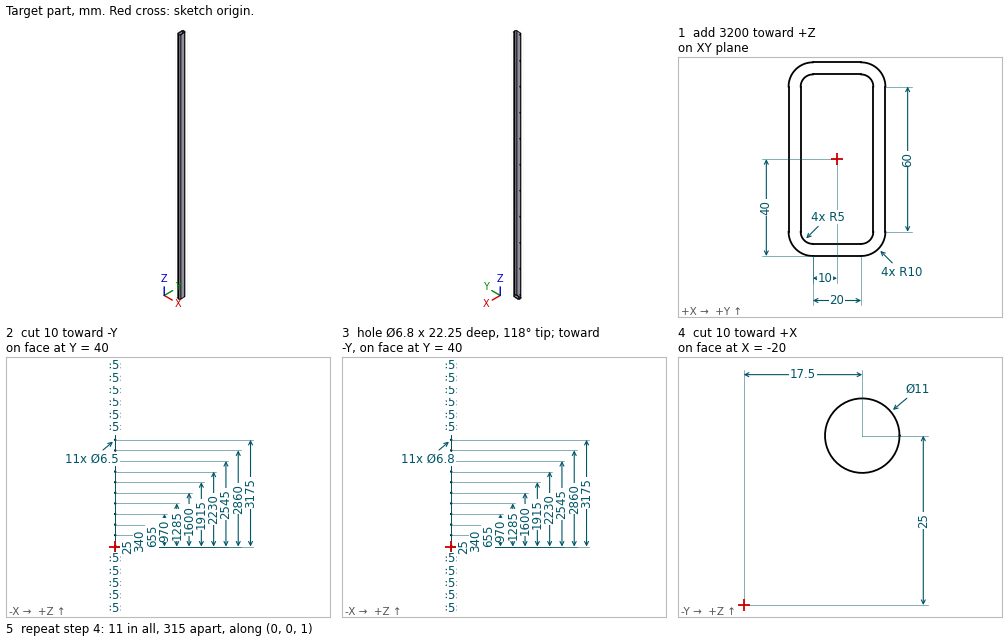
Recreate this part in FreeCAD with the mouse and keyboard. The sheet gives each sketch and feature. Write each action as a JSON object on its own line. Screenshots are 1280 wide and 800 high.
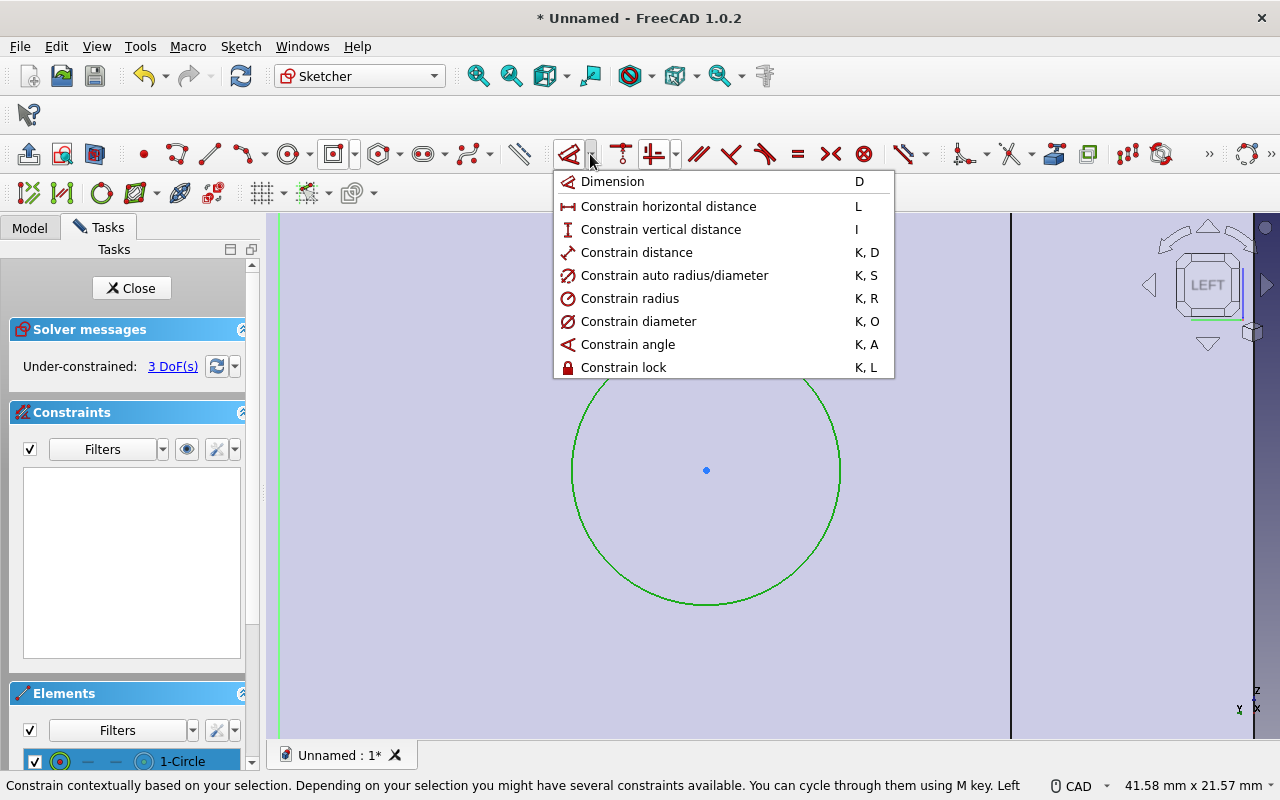
{"action": "left_click", "coordinate": [724, 322]}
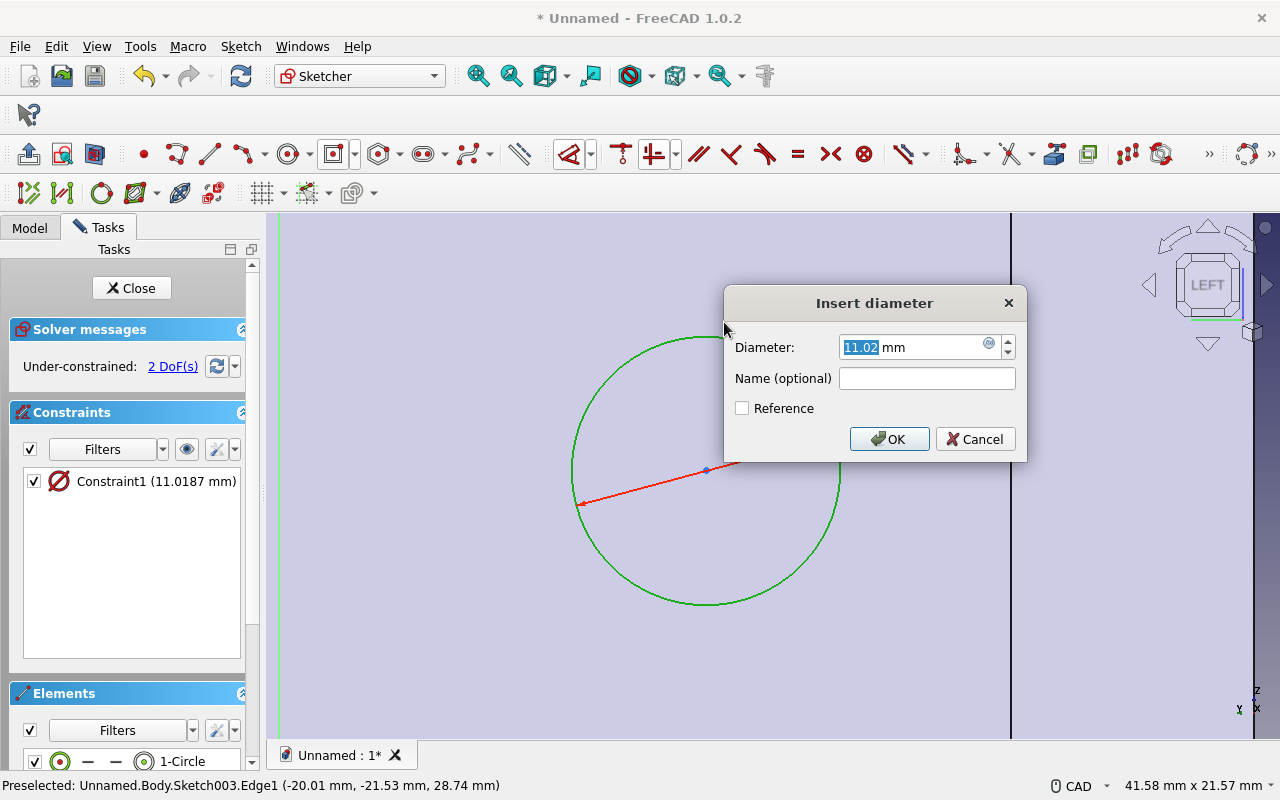
{"action": "type", "text": "11"}
{"action": "key", "text": "Return"}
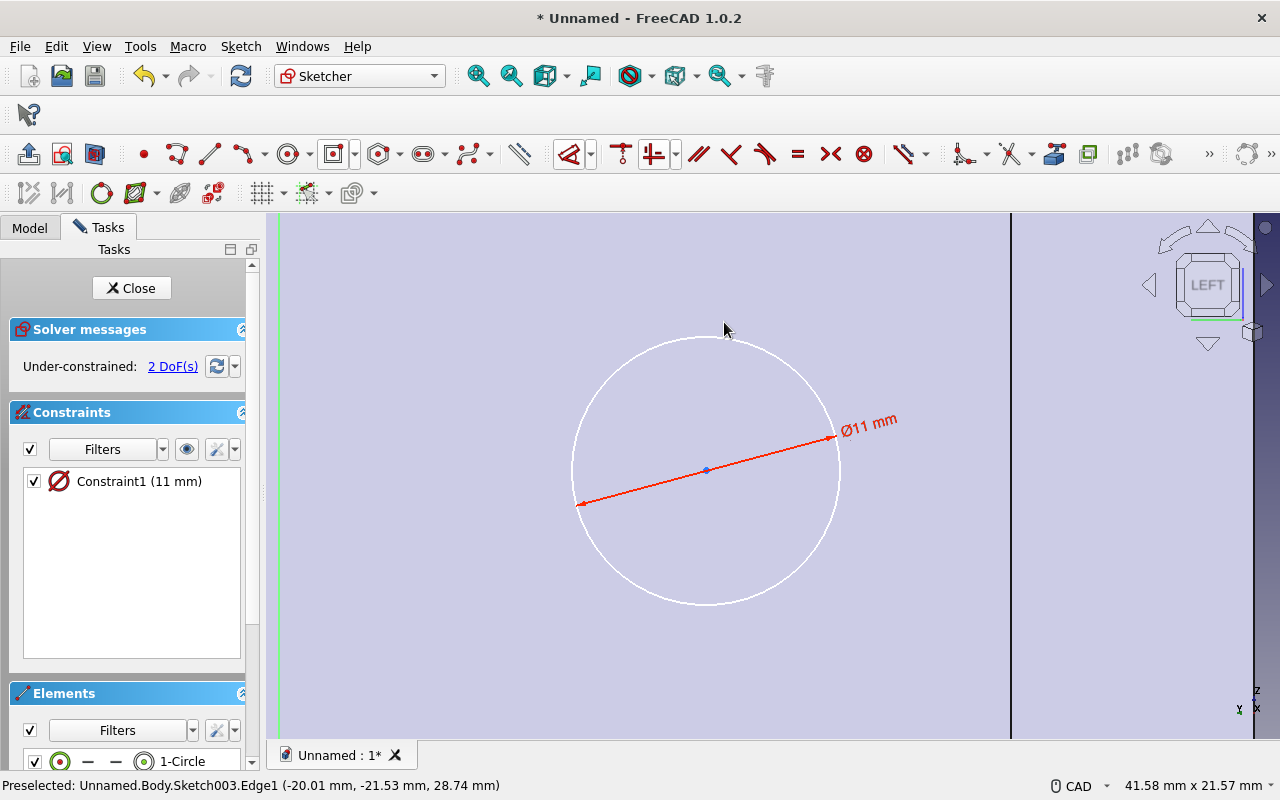
{"action": "left_click", "coordinate": [706, 471]}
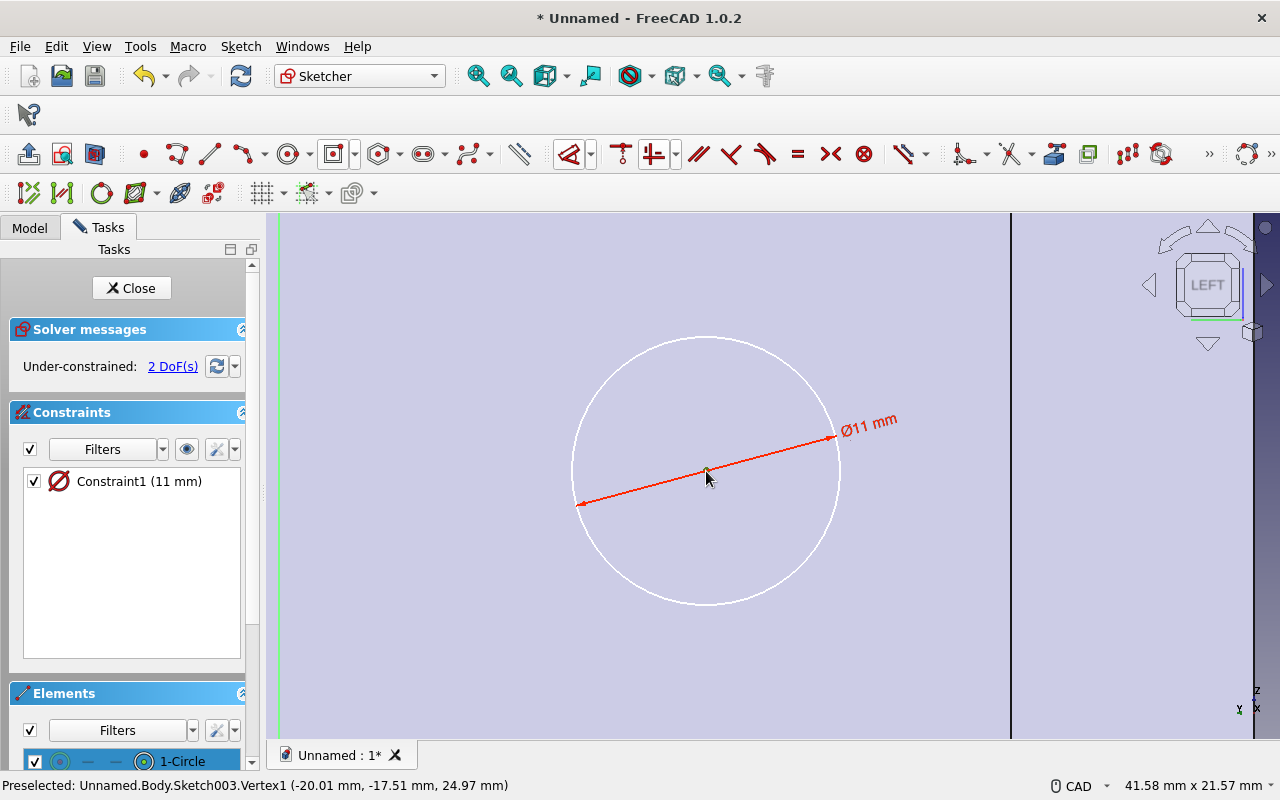
{"action": "key", "text": "i"}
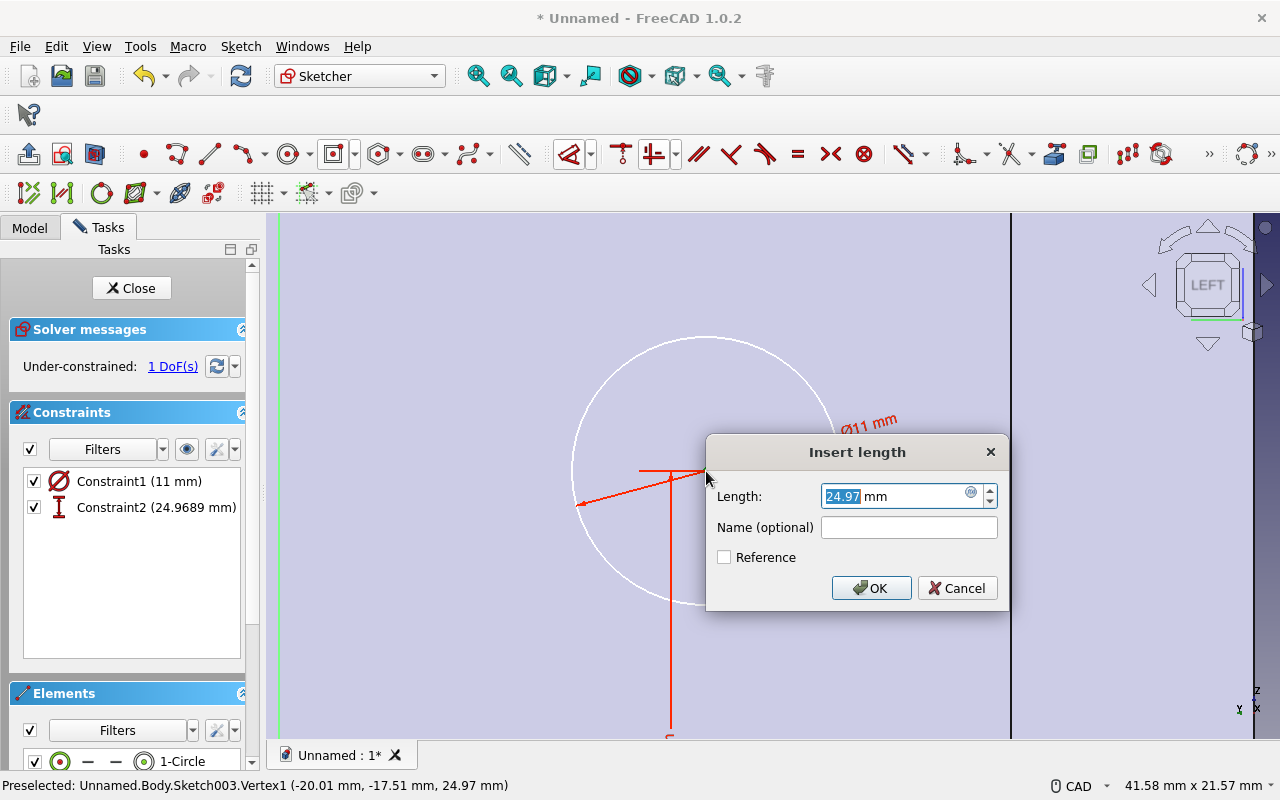
{"action": "type", "text": "25"}
{"action": "key", "text": "Return"}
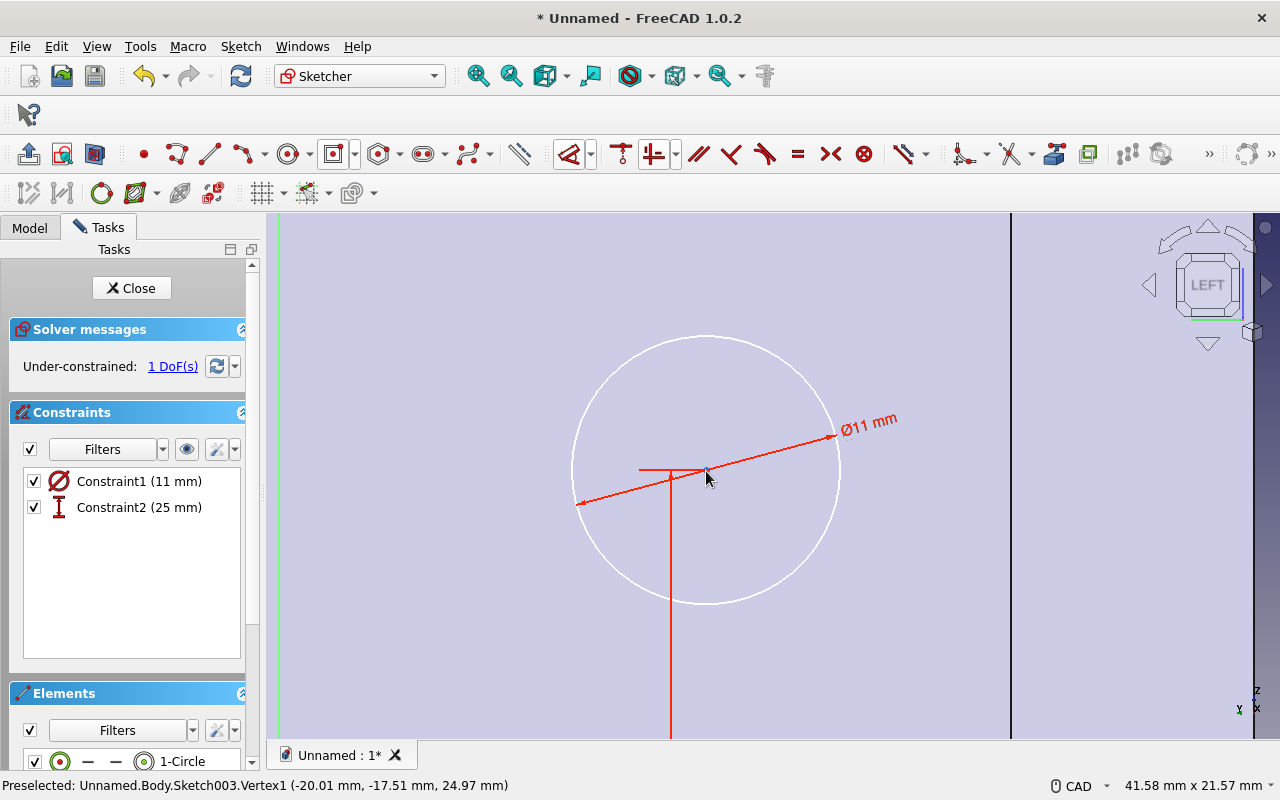
{"action": "left_click", "coordinate": [706, 470]}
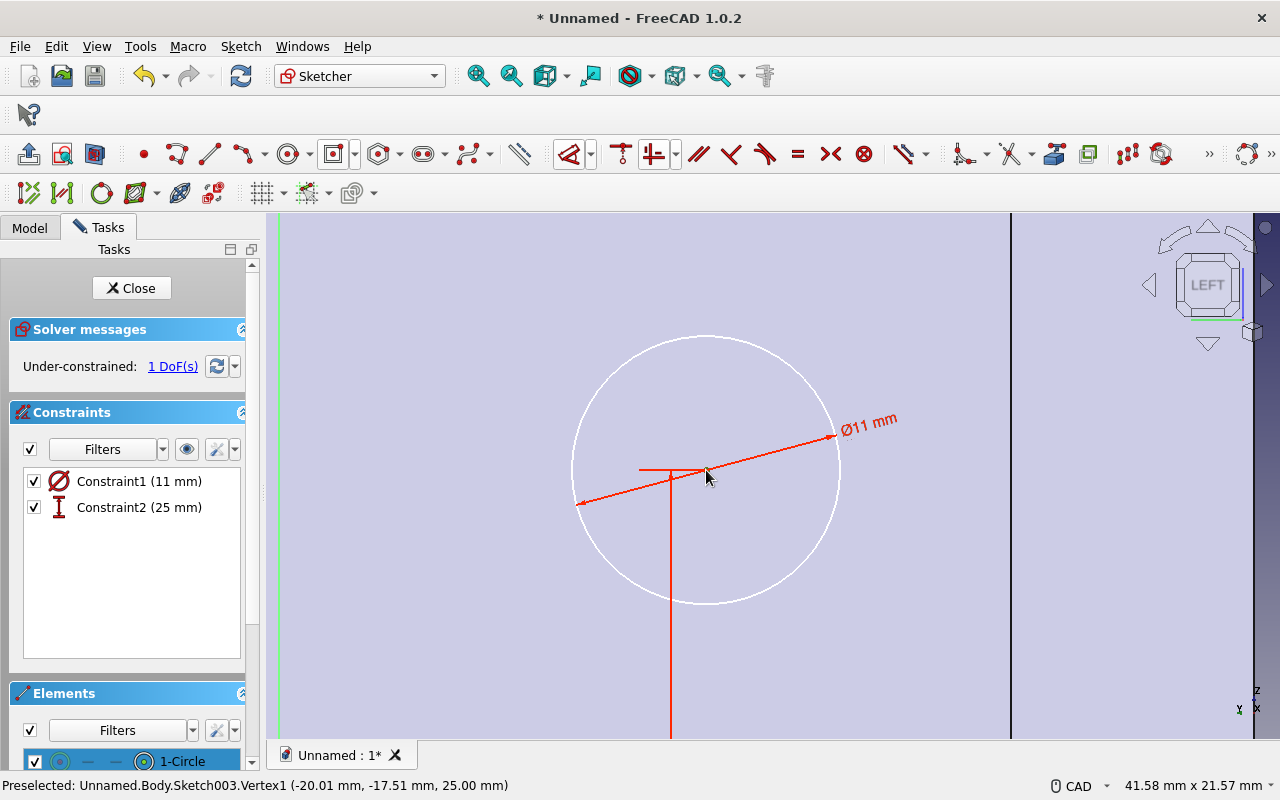
{"action": "left_click", "coordinate": [590, 154]}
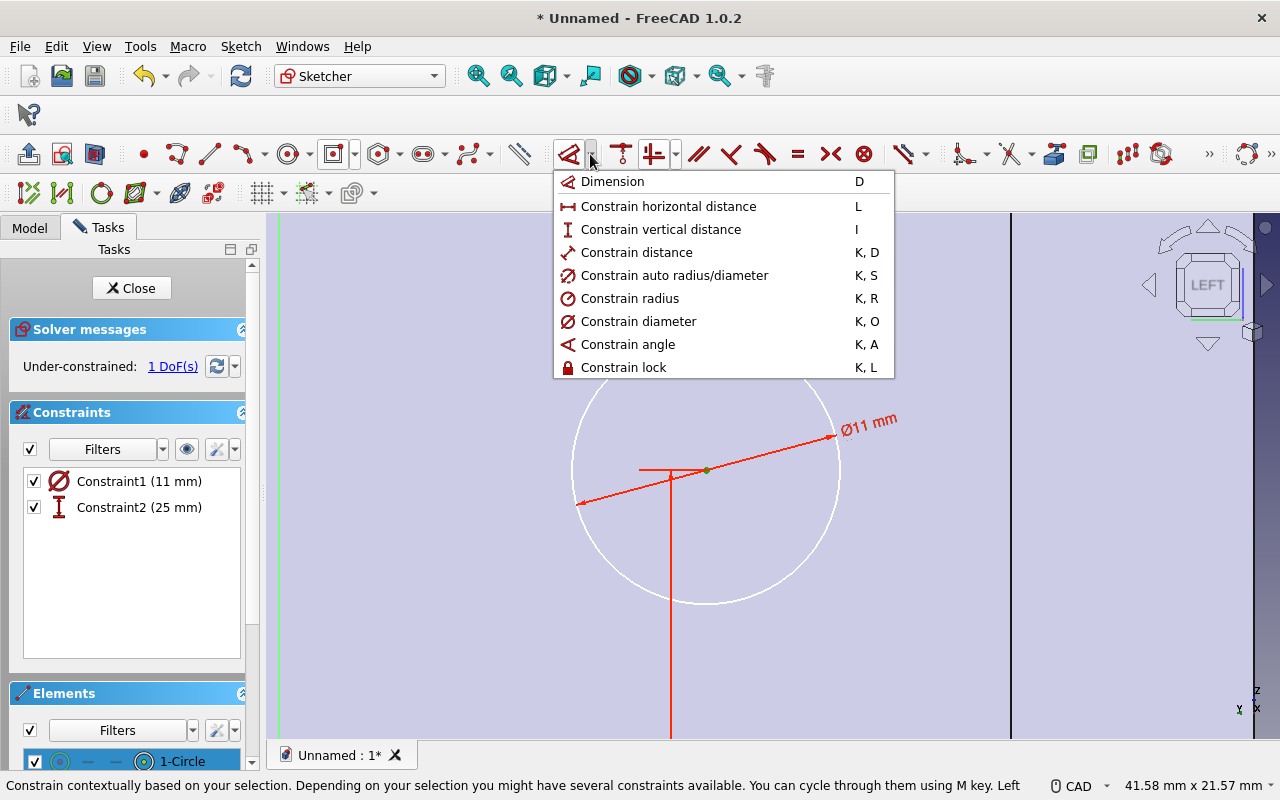
{"action": "left_click", "coordinate": [724, 206]}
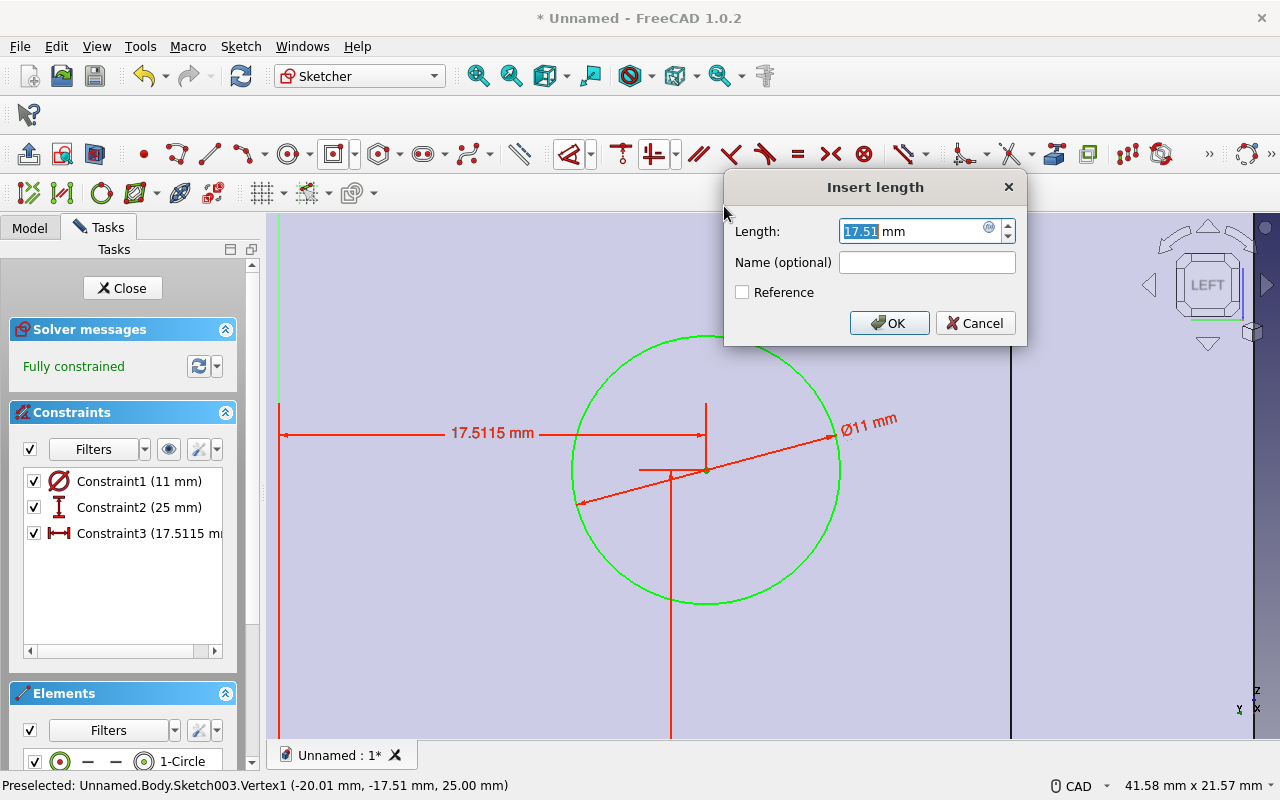
{"action": "type", "text": "17.5"}
{"action": "key", "text": "Return"}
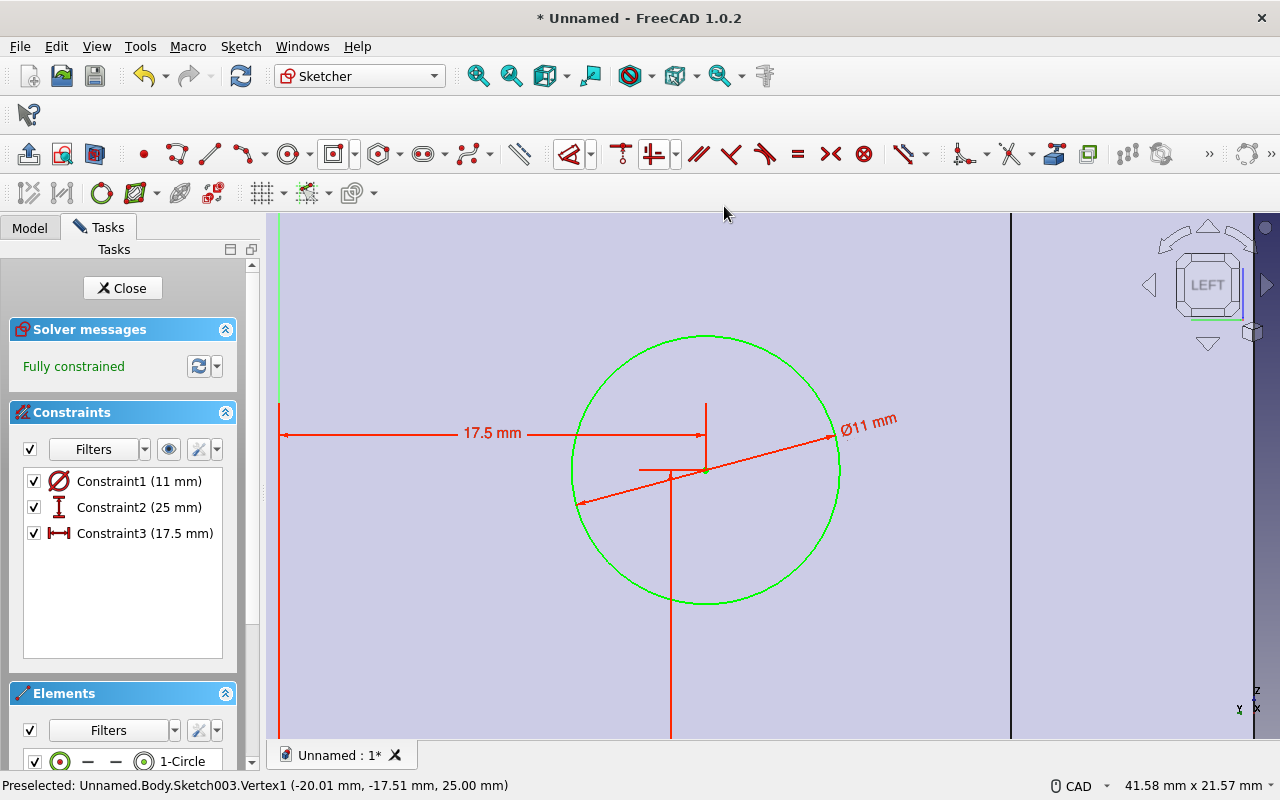
{"action": "left_click", "coordinate": [123, 288]}